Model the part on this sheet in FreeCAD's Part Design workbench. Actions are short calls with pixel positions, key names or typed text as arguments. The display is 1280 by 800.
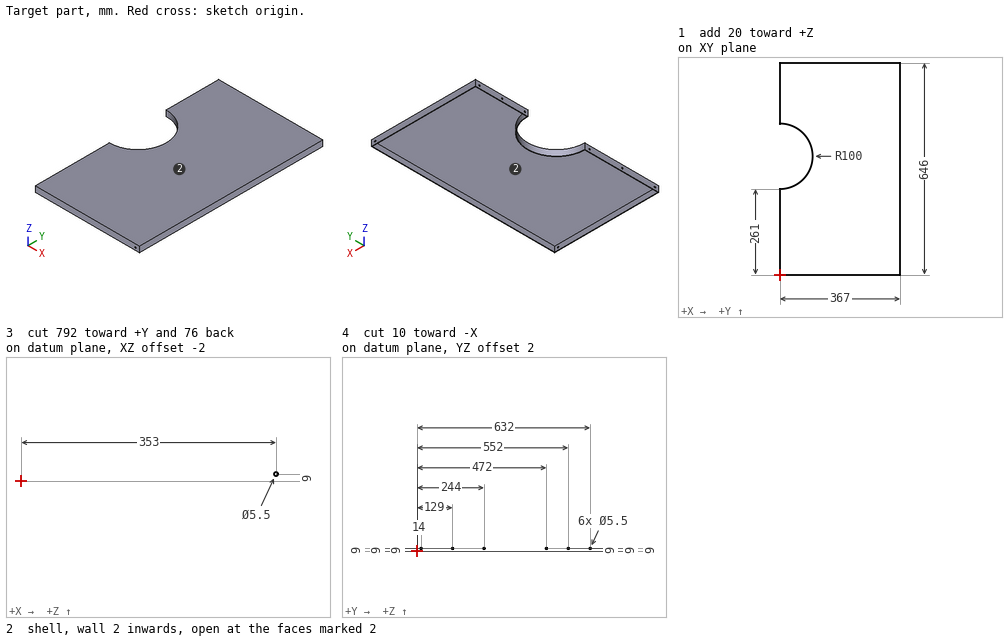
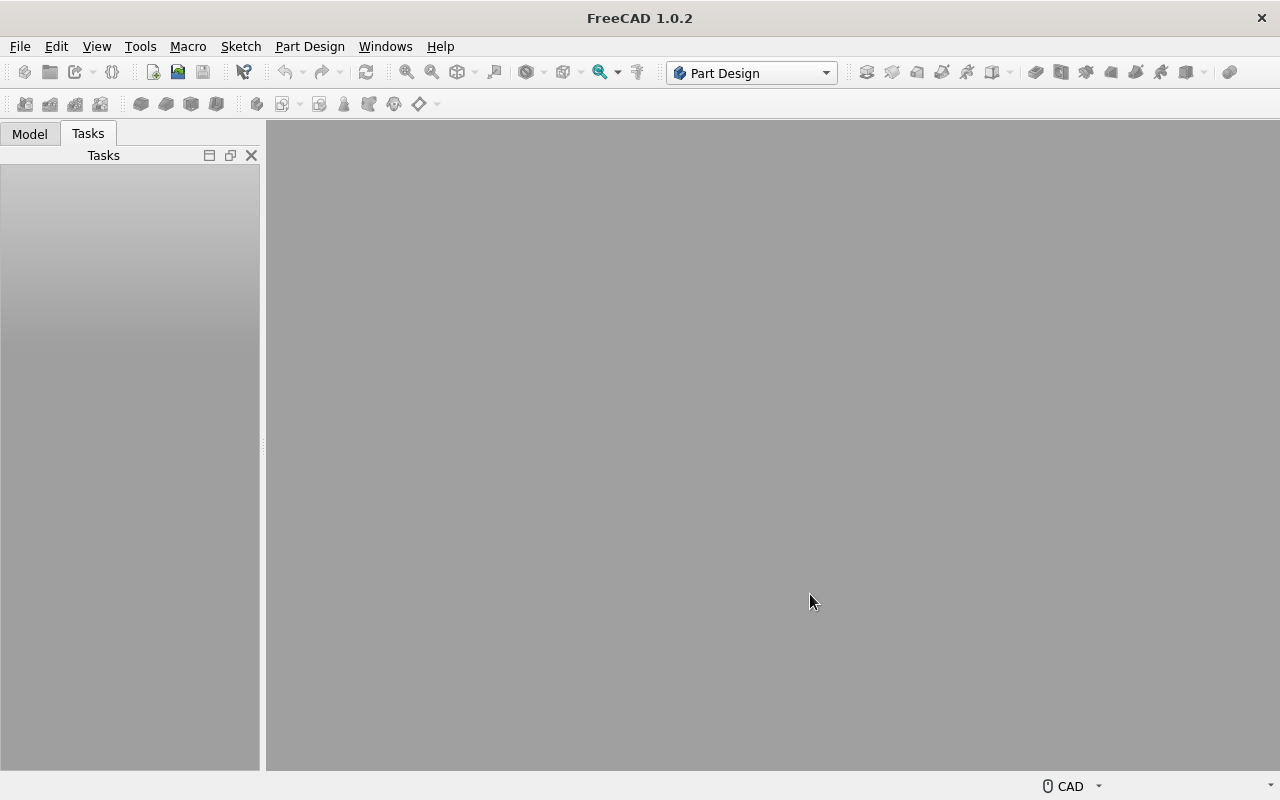
click(153, 72)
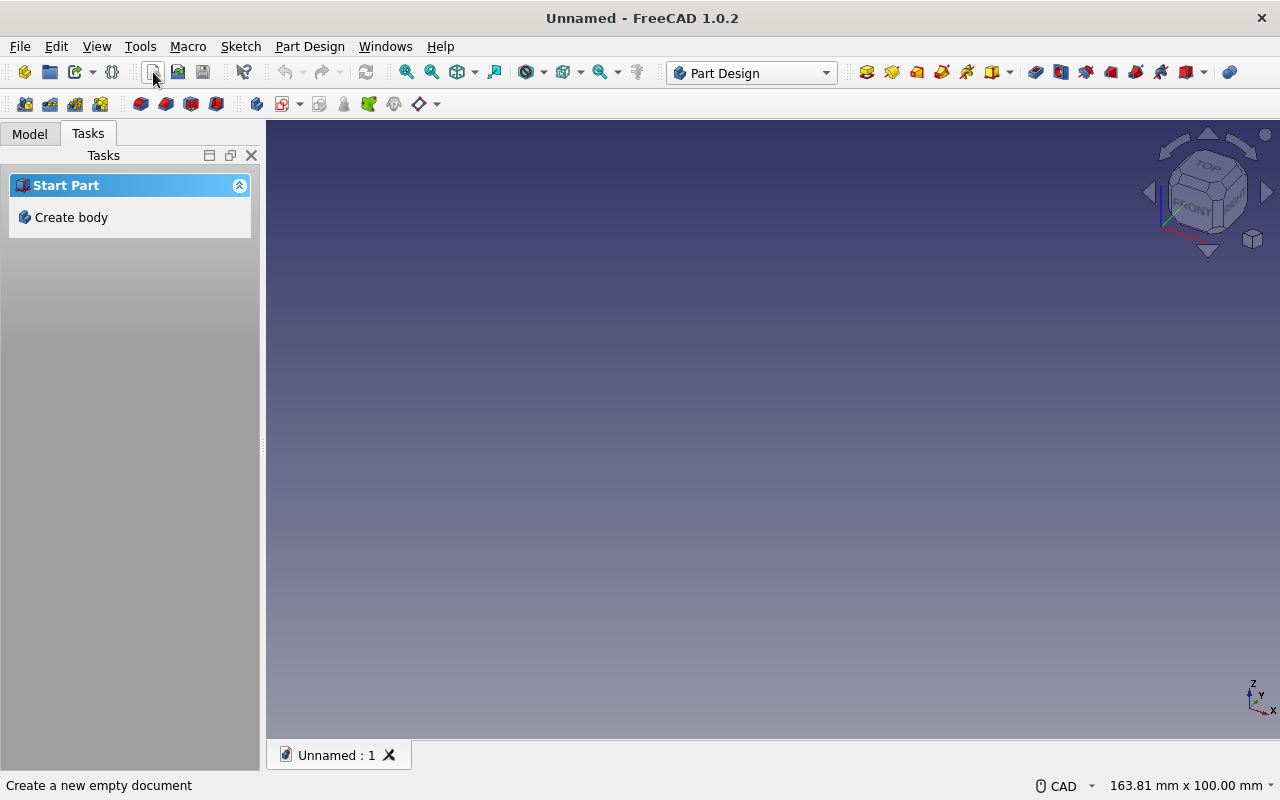
click(282, 104)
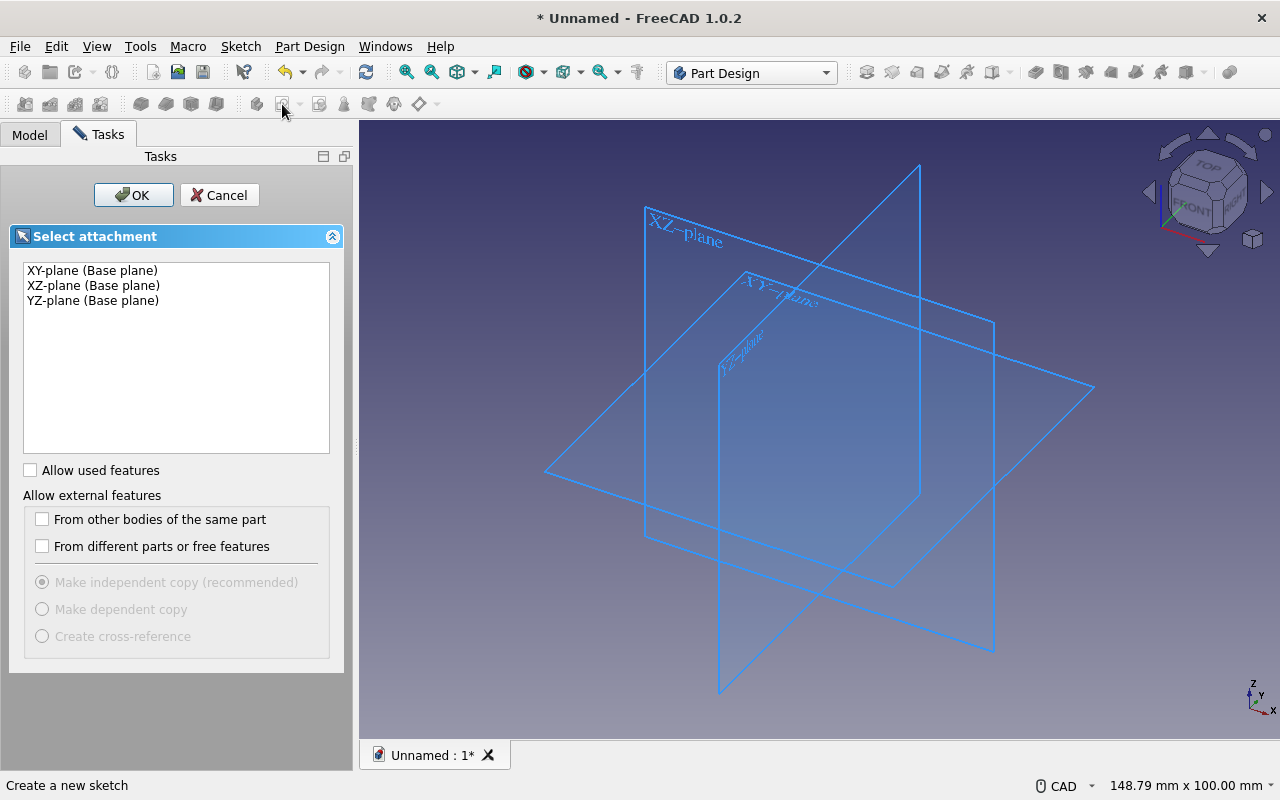
click(84, 270)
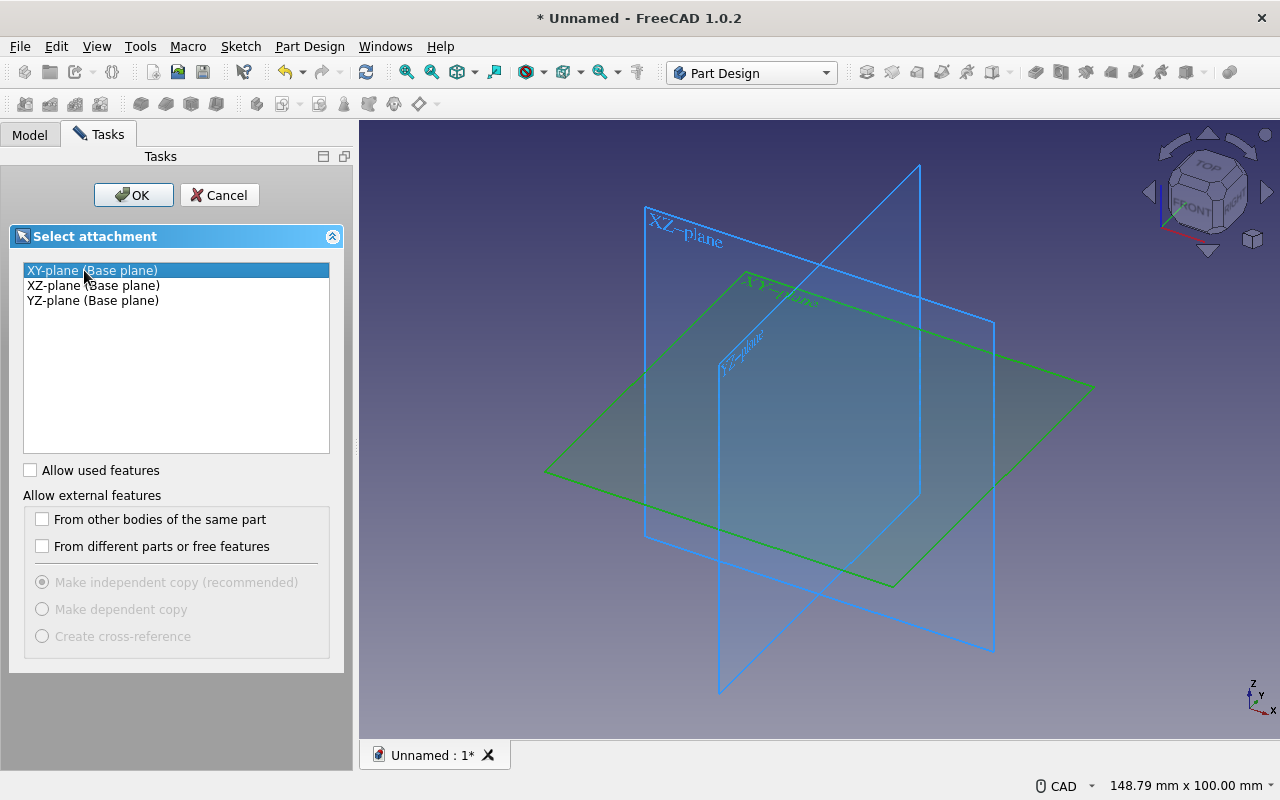
click(134, 195)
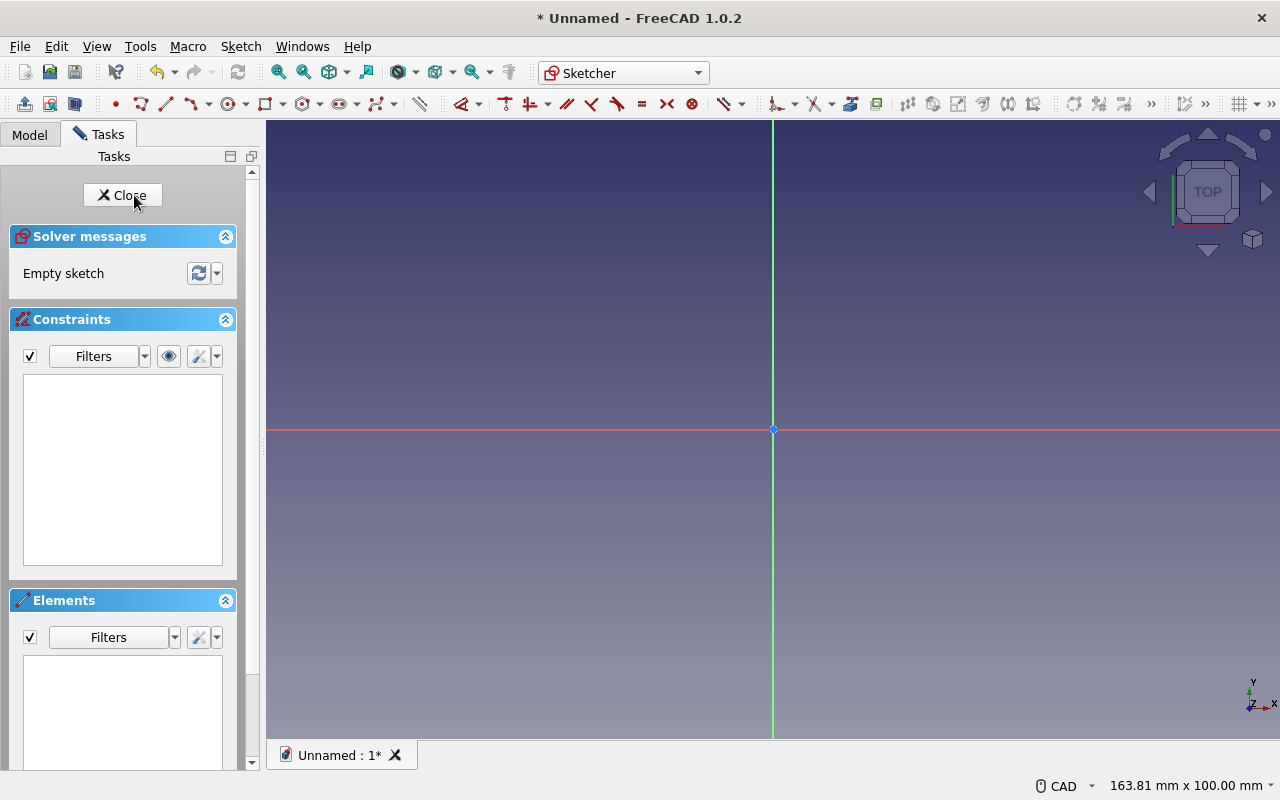
scroll(584, 629, down, 12)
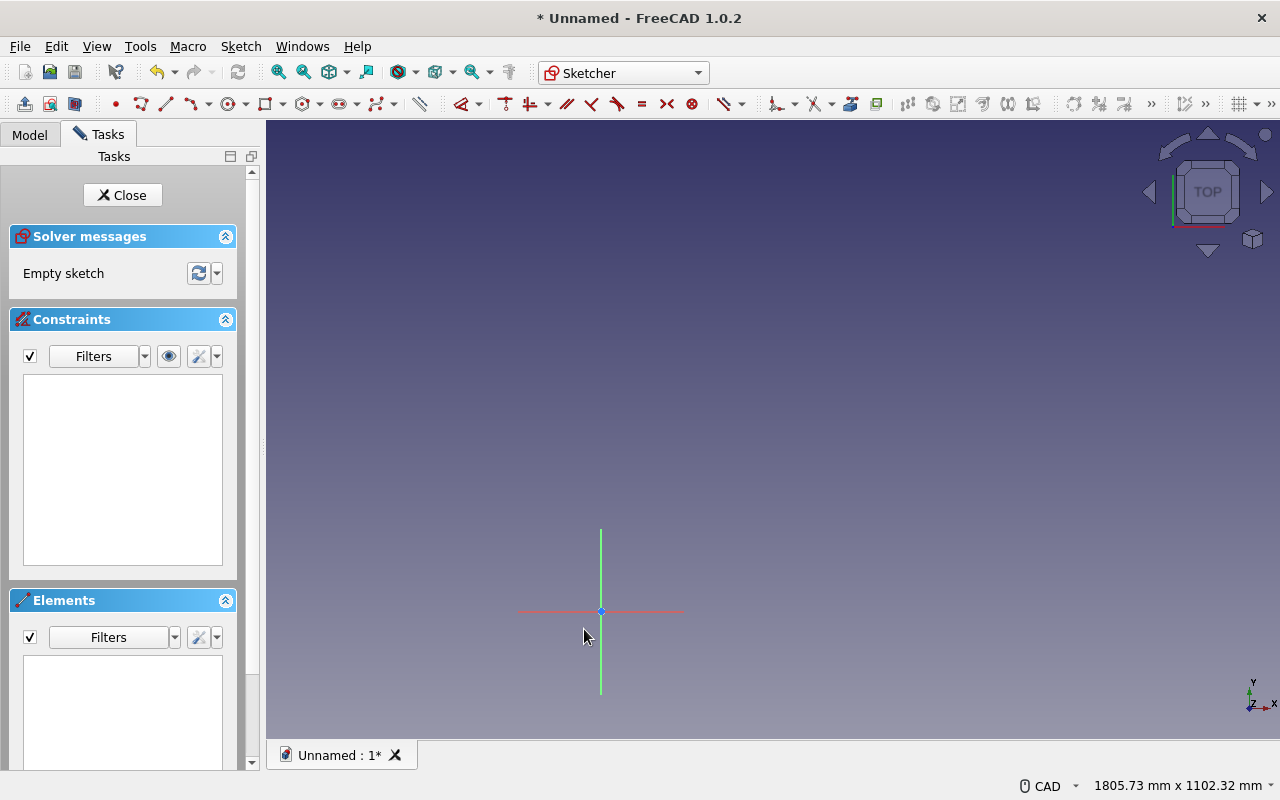
click(141, 104)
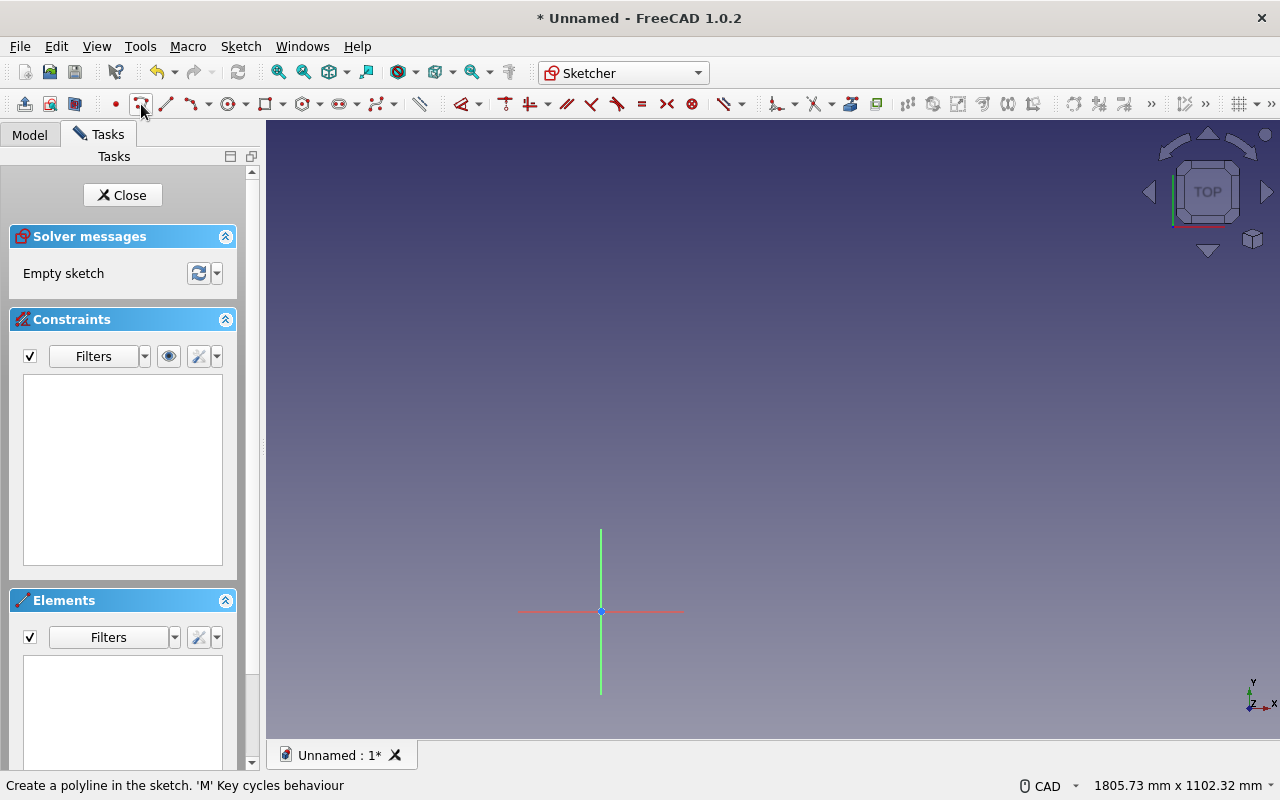
click(601, 465)
click(601, 612)
click(808, 603)
click(808, 249)
click(601, 249)
click(610, 353)
right_click(610, 353)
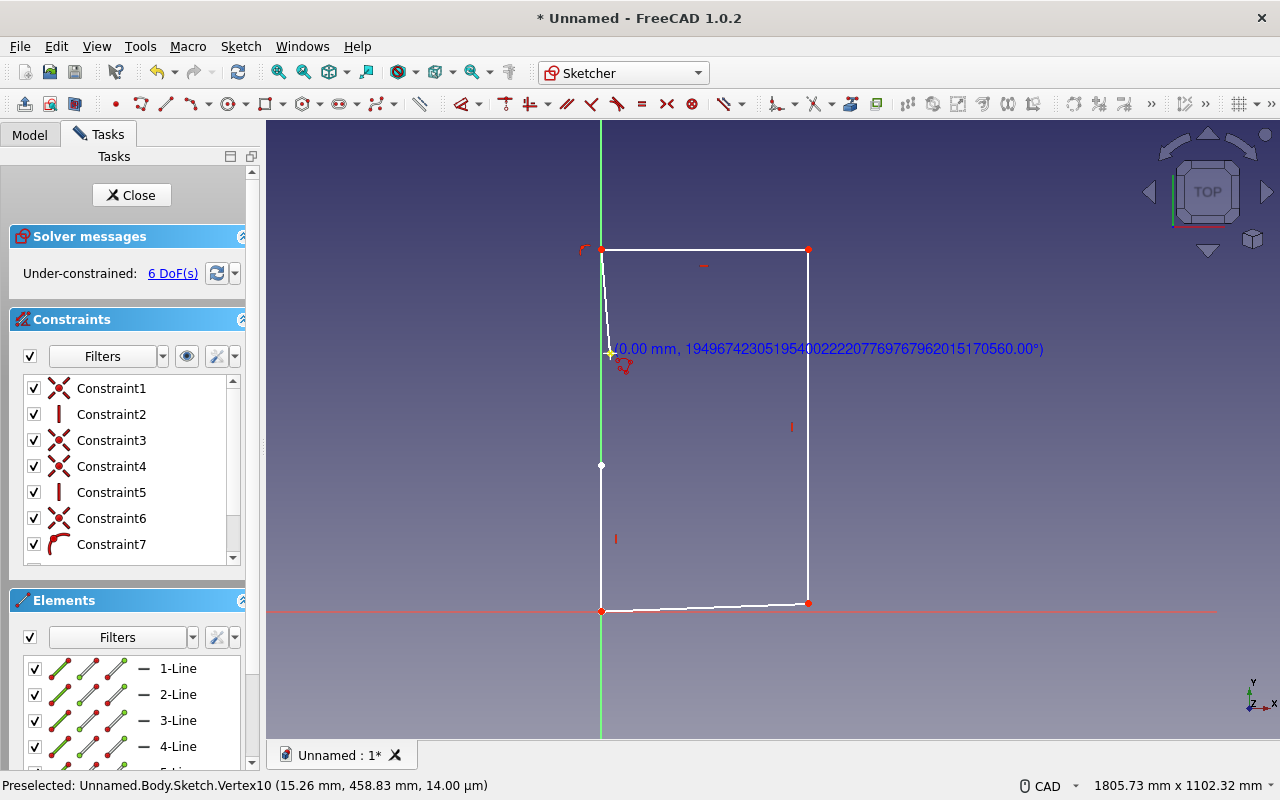
click(190, 104)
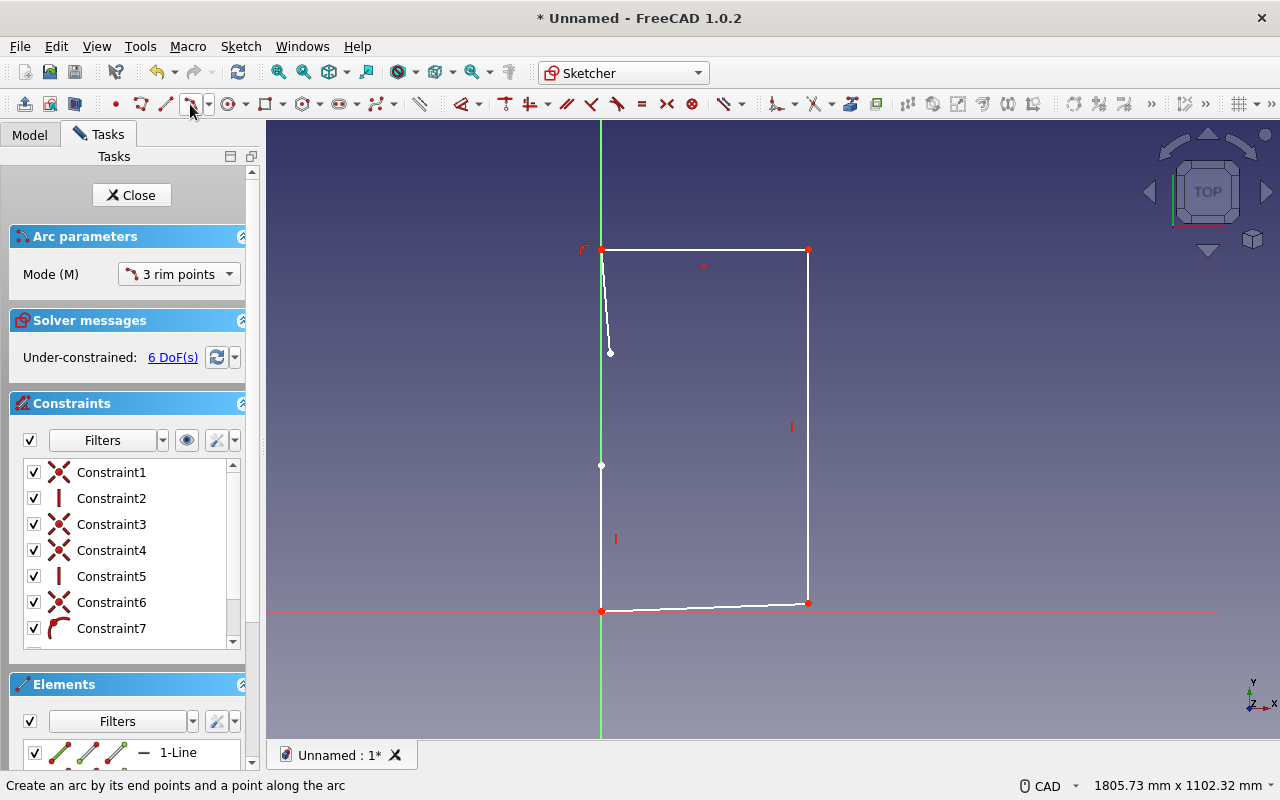
click(610, 354)
click(601, 466)
click(658, 409)
key(Escape)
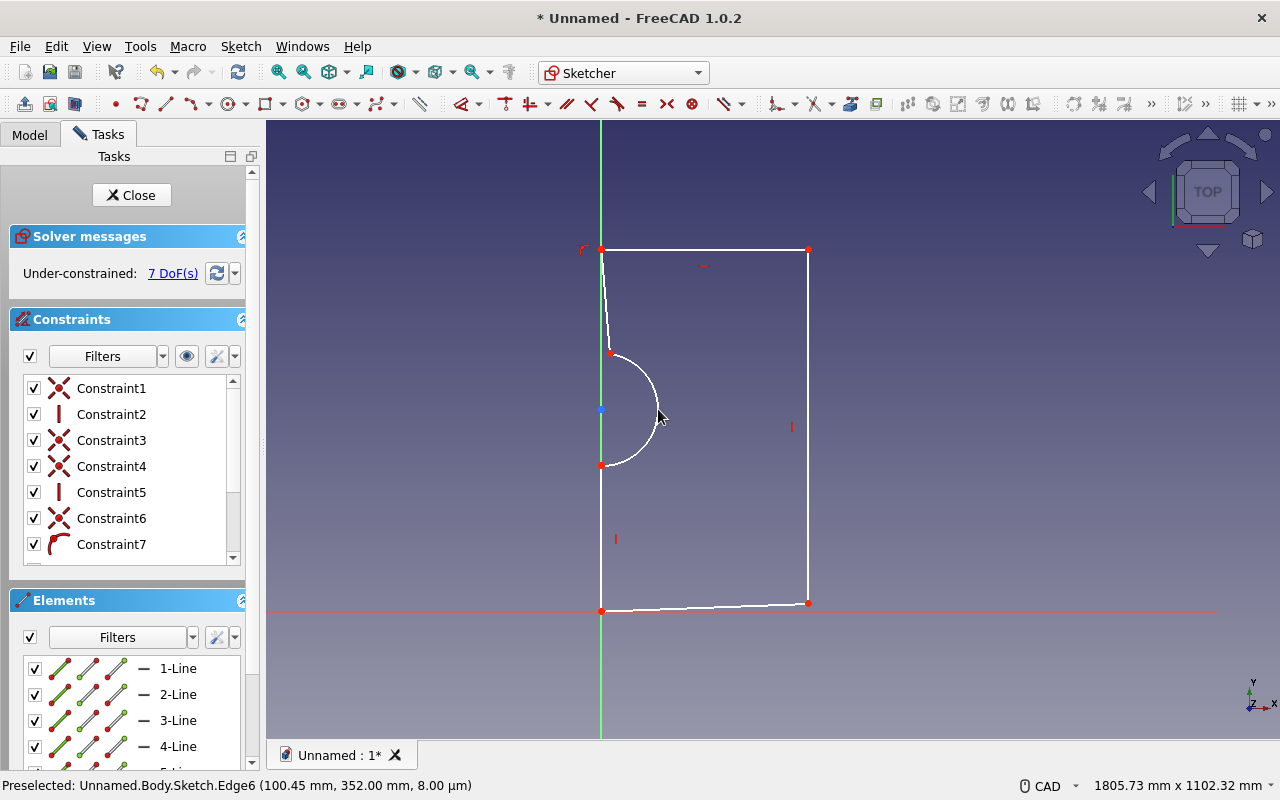
click(663, 609)